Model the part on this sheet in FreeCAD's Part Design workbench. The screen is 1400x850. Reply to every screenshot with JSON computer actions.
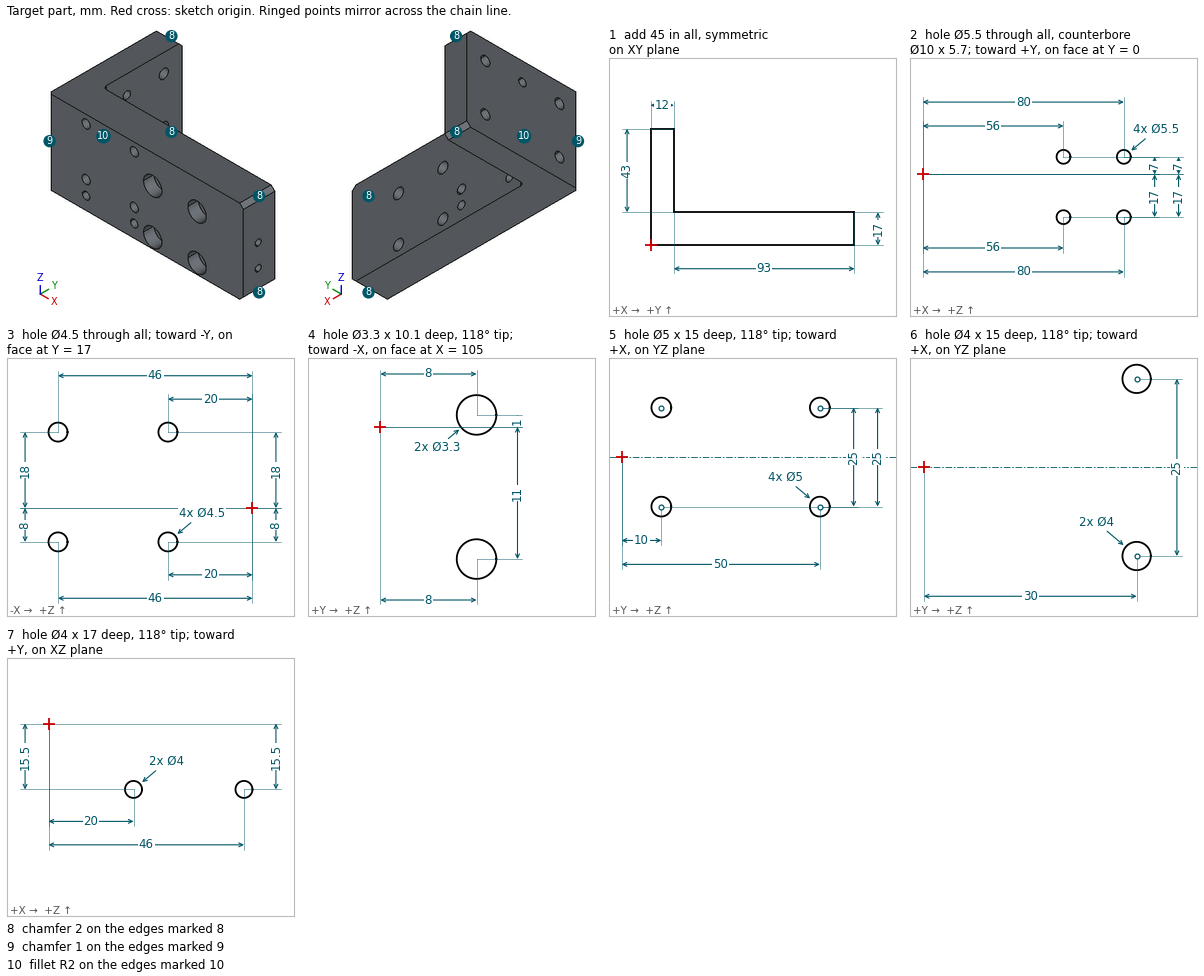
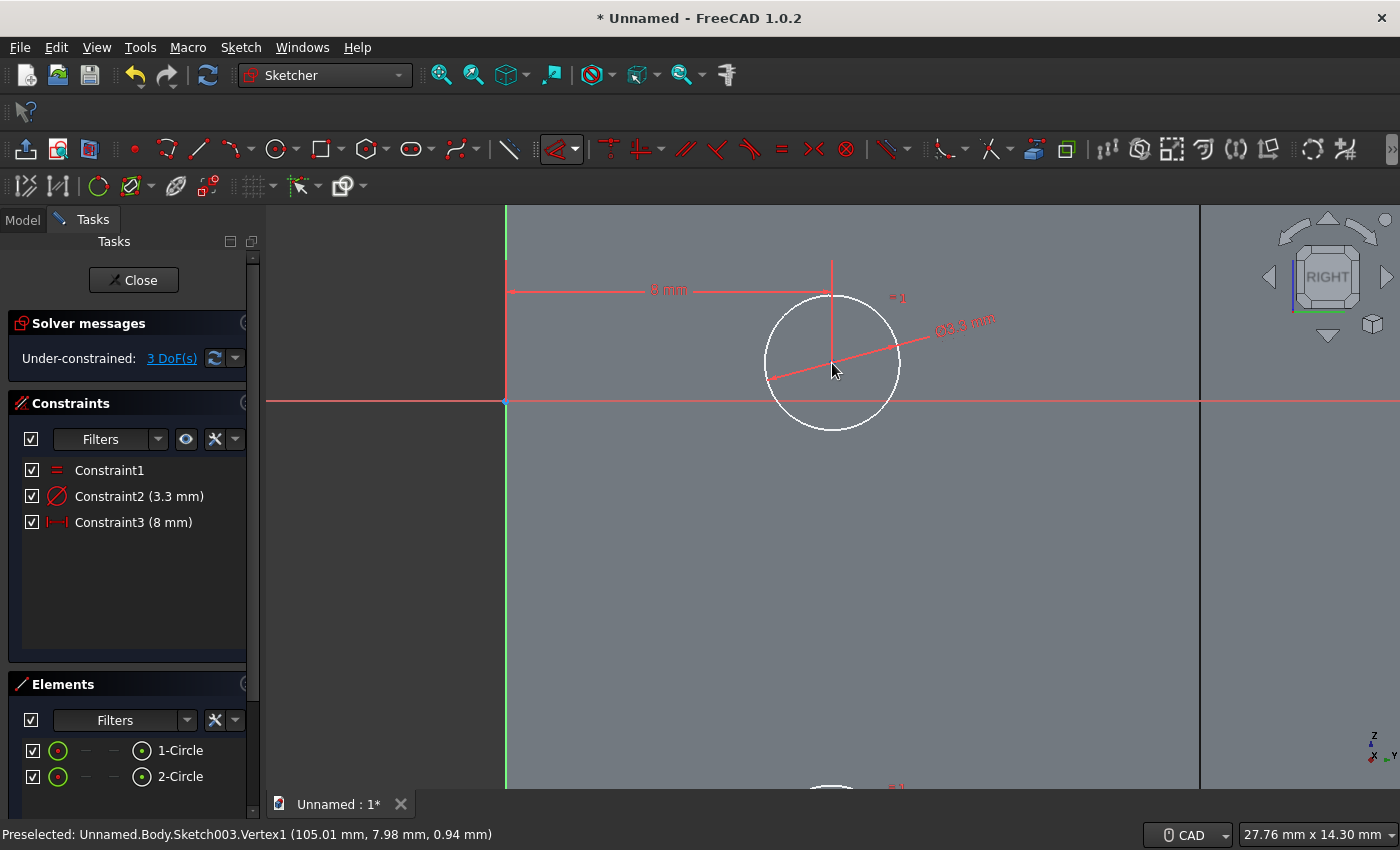
{"action": "left_click", "coordinate": [832, 363]}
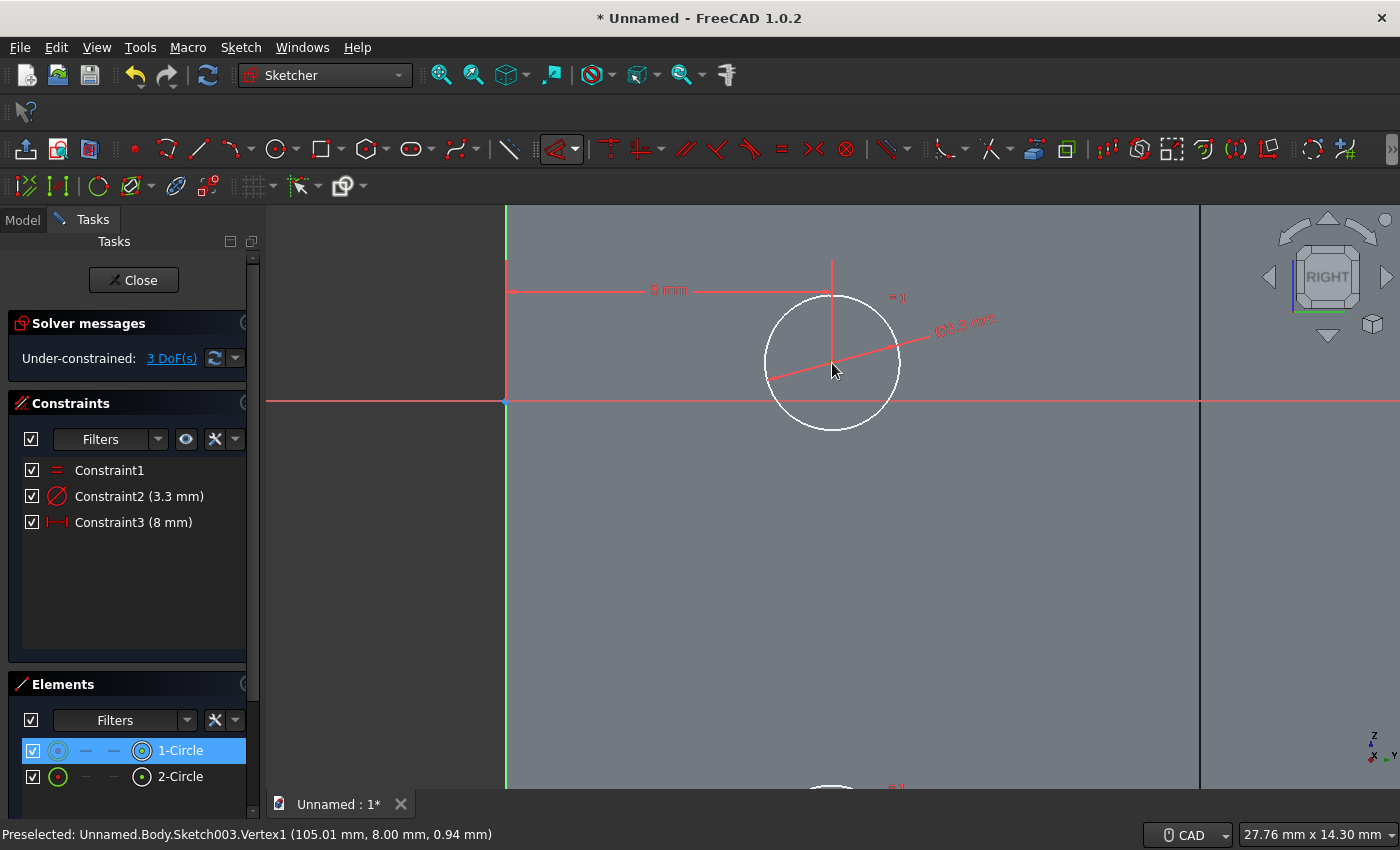
{"action": "key", "text": "i"}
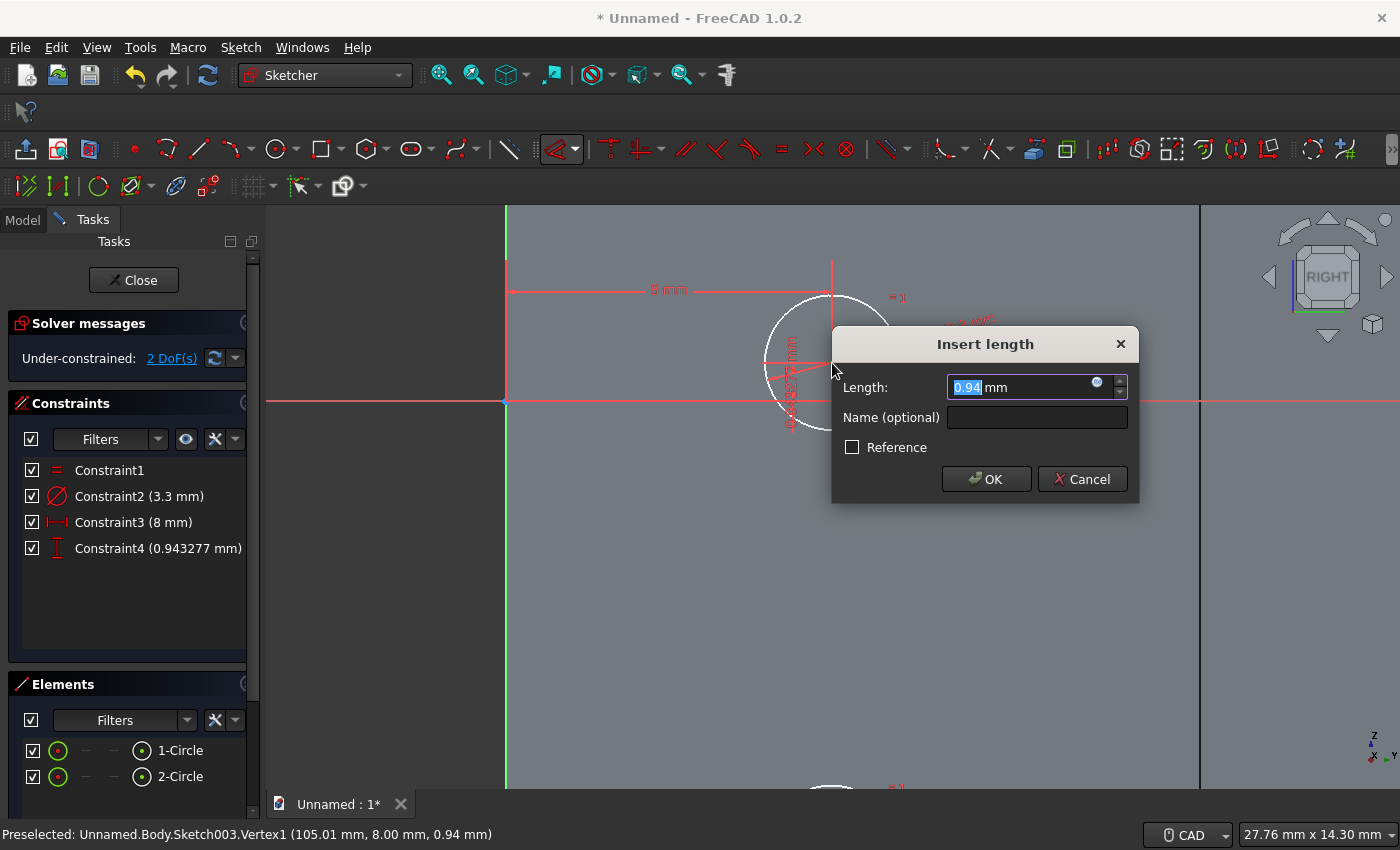
{"action": "type", "text": "1"}
{"action": "key", "text": "Return"}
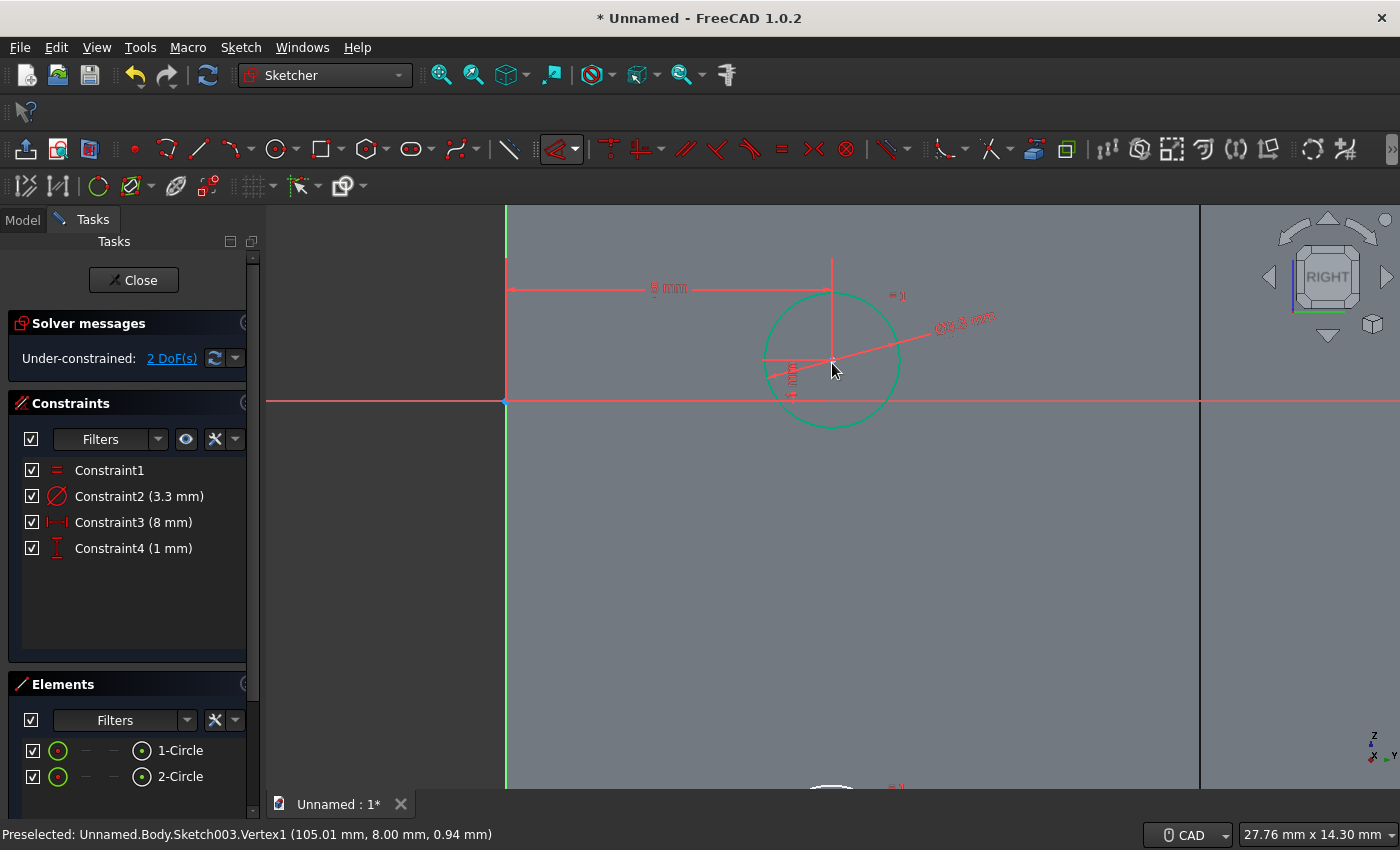
{"action": "scroll", "coordinate": [840, 365], "scroll_direction": "down", "scroll_amount": 3}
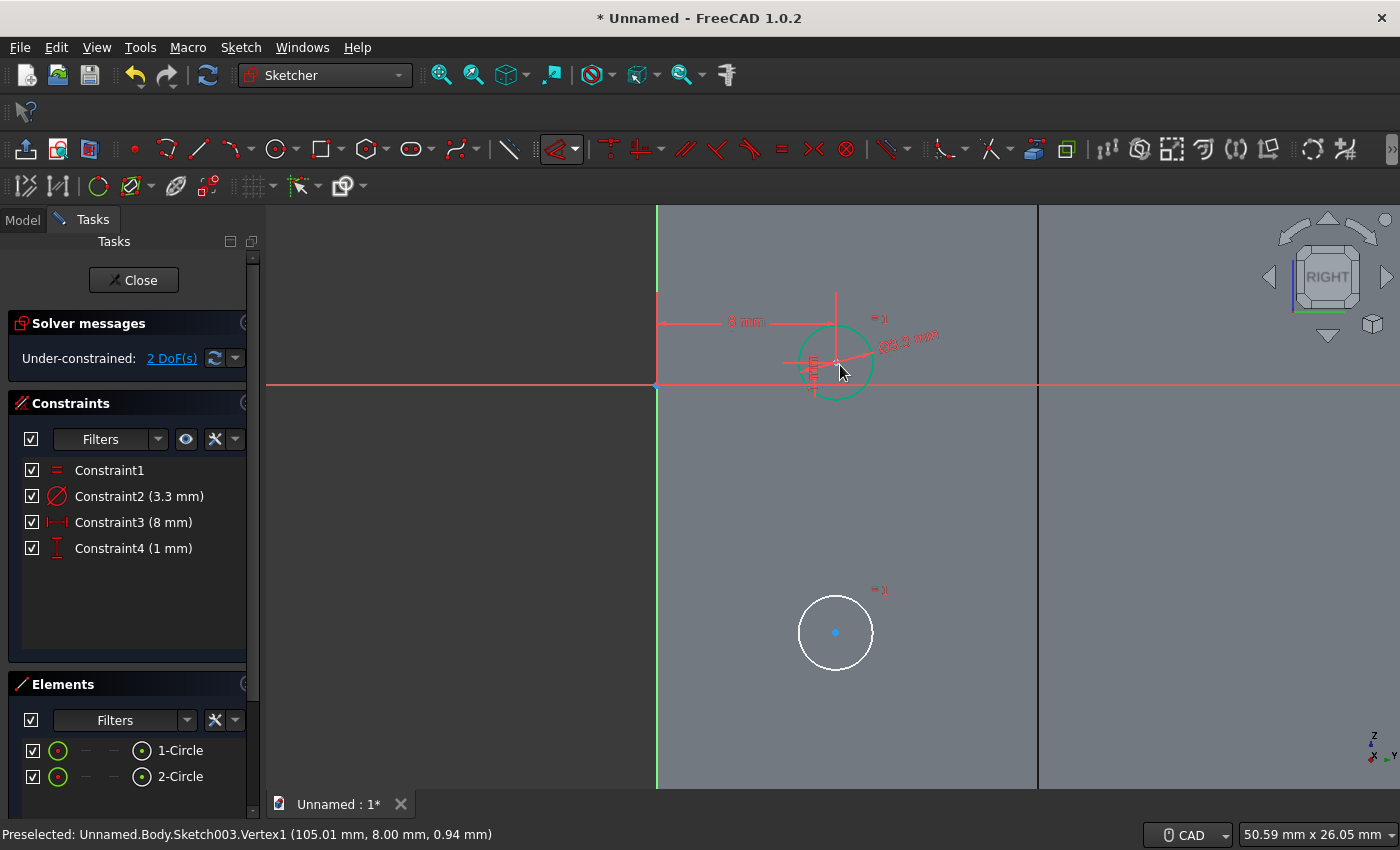
{"action": "left_click", "coordinate": [836, 633]}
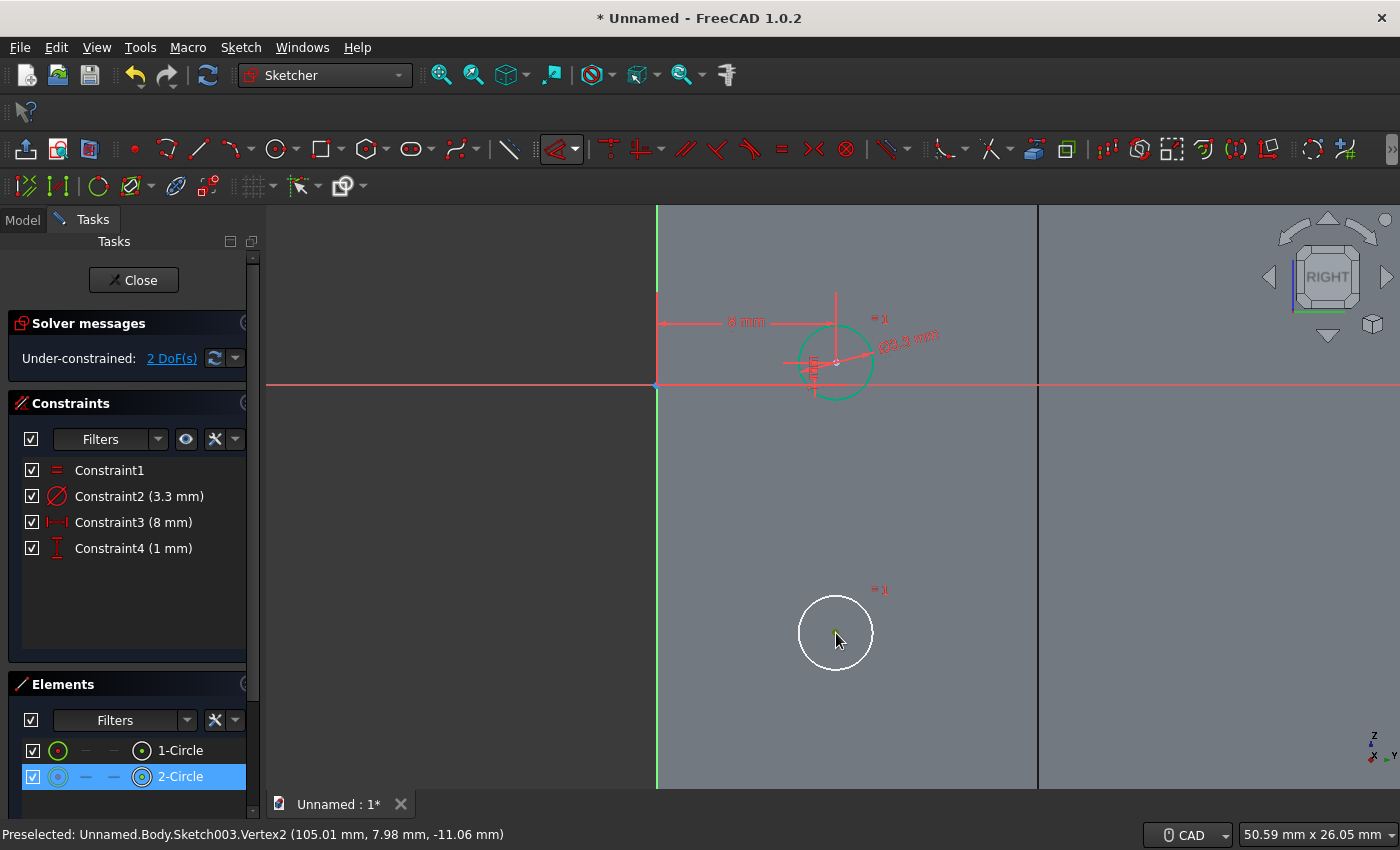
{"action": "key", "text": "l"}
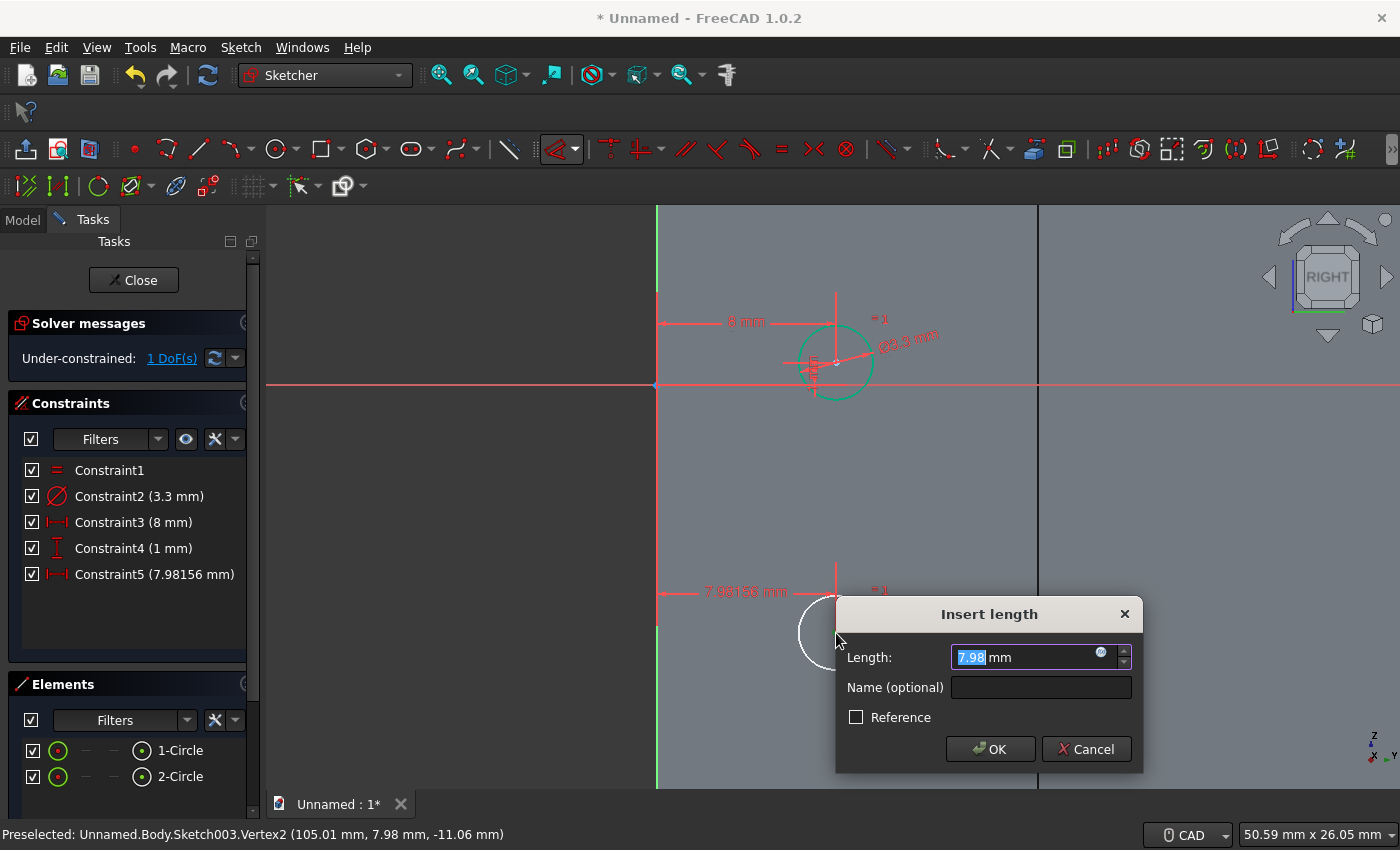
{"action": "type", "text": "8"}
{"action": "key", "text": "Return"}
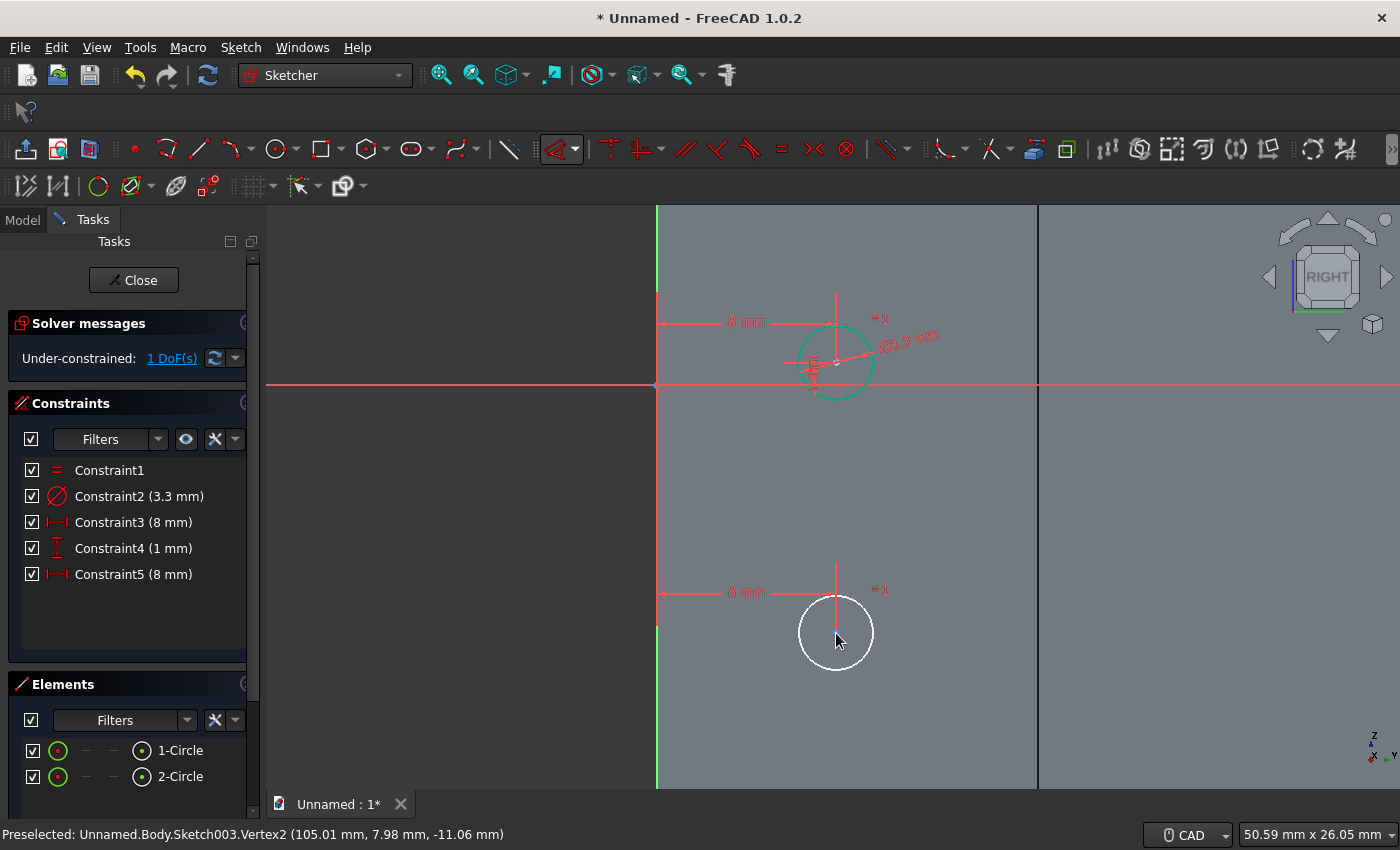
{"action": "left_click", "coordinate": [836, 633]}